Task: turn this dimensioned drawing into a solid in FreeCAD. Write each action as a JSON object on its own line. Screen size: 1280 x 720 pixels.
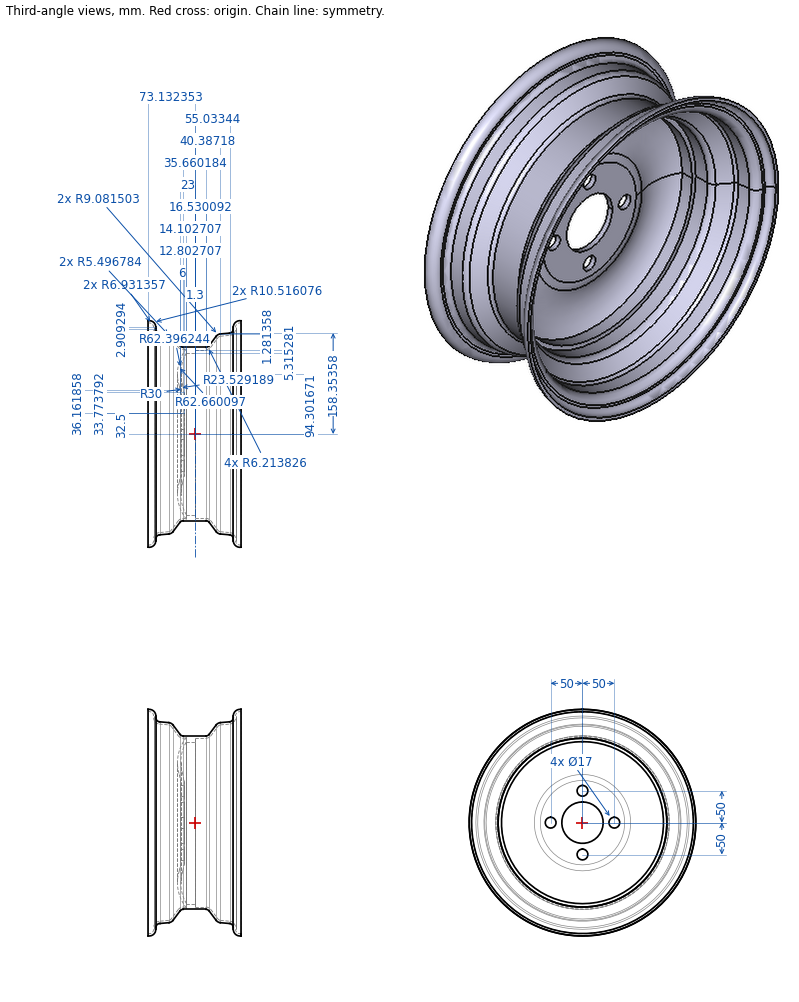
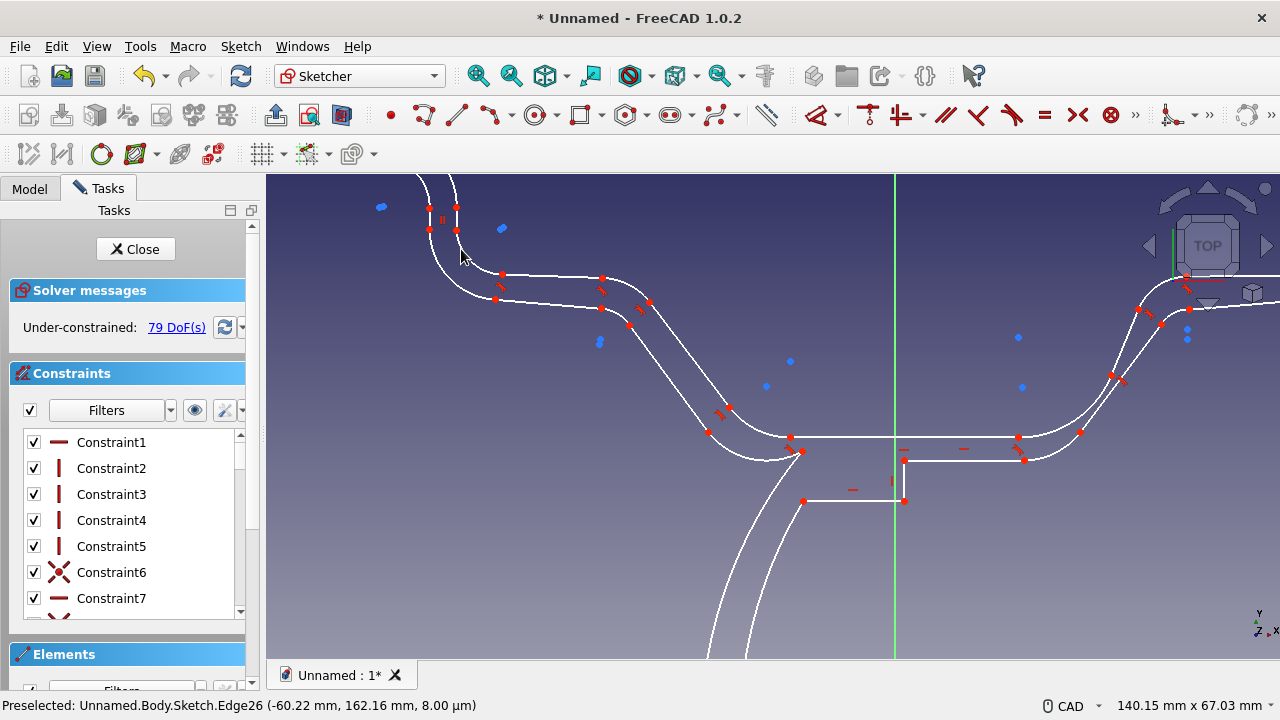
{"action": "scroll", "coordinate": [457, 219], "scroll_direction": "up", "scroll_amount": 2}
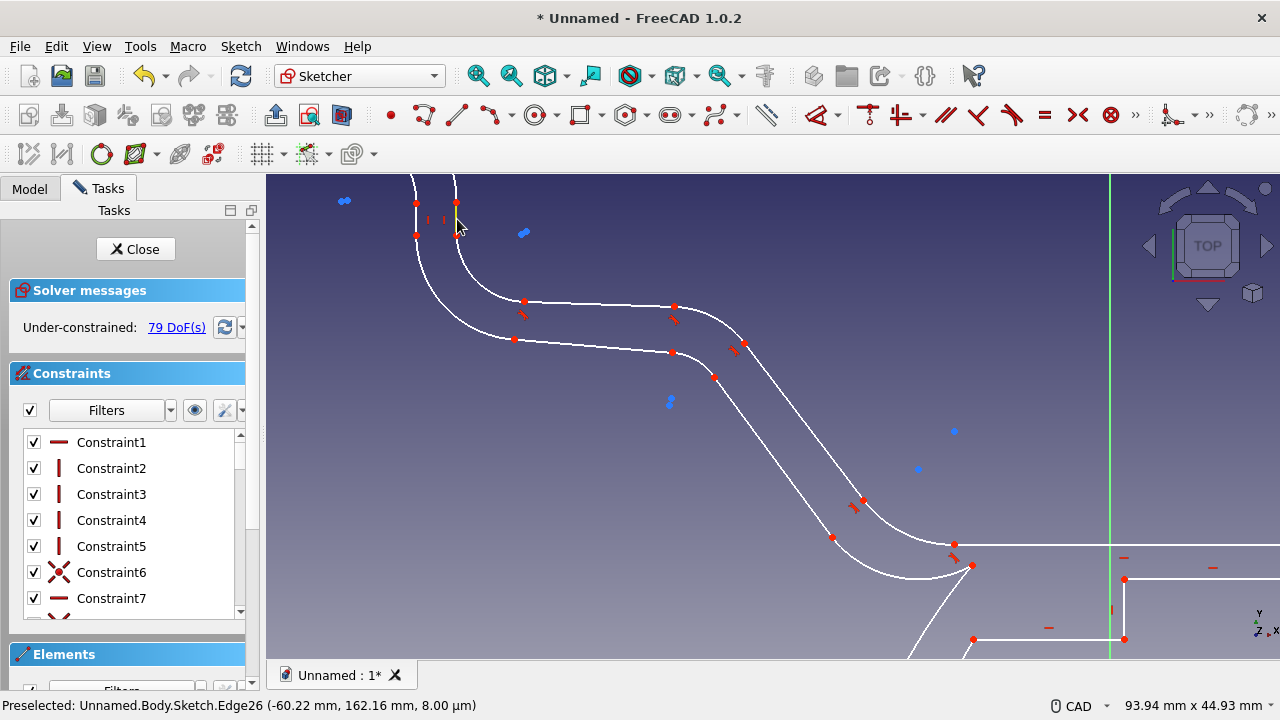
{"action": "left_click", "coordinate": [456, 219]}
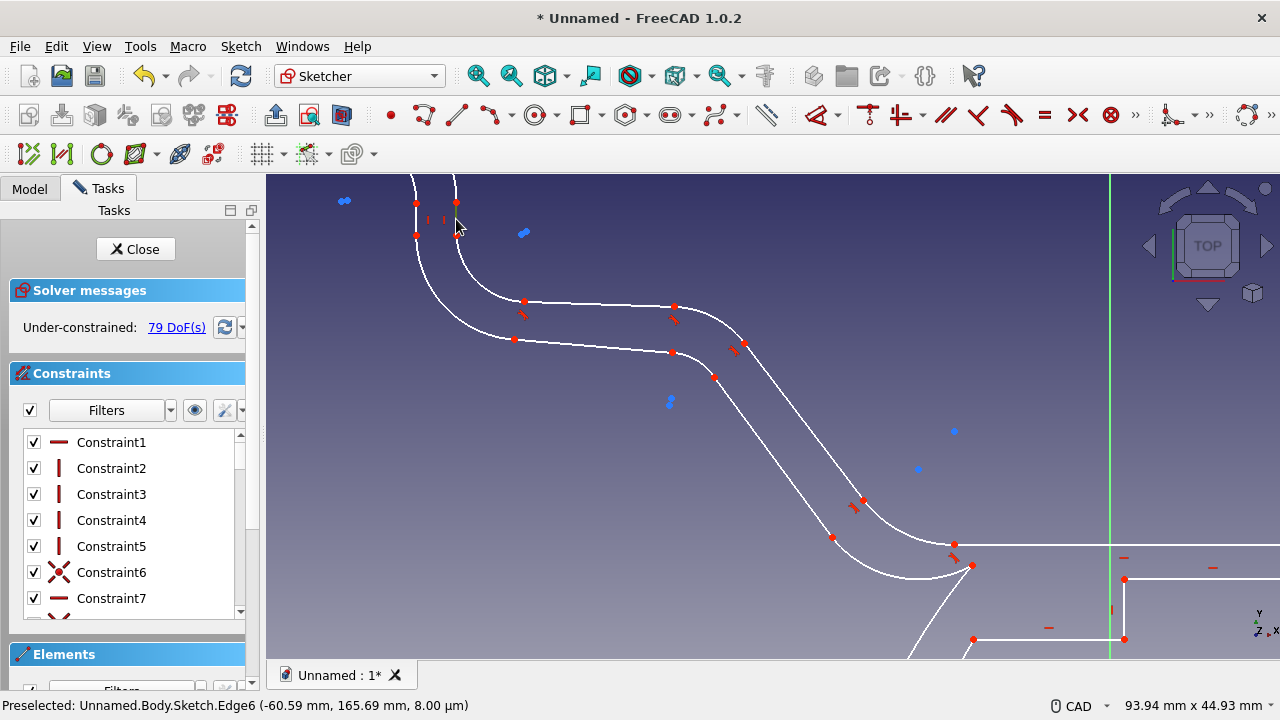
{"action": "left_click", "coordinate": [465, 265]}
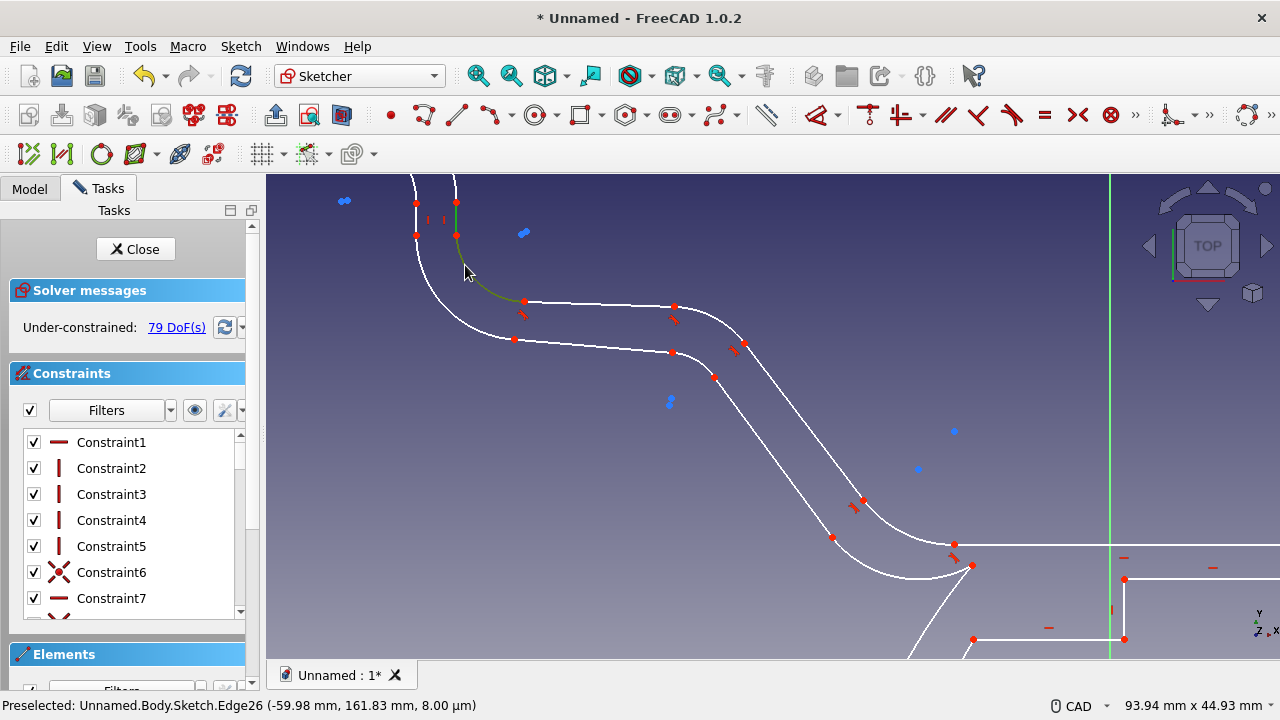
{"action": "key", "text": "t"}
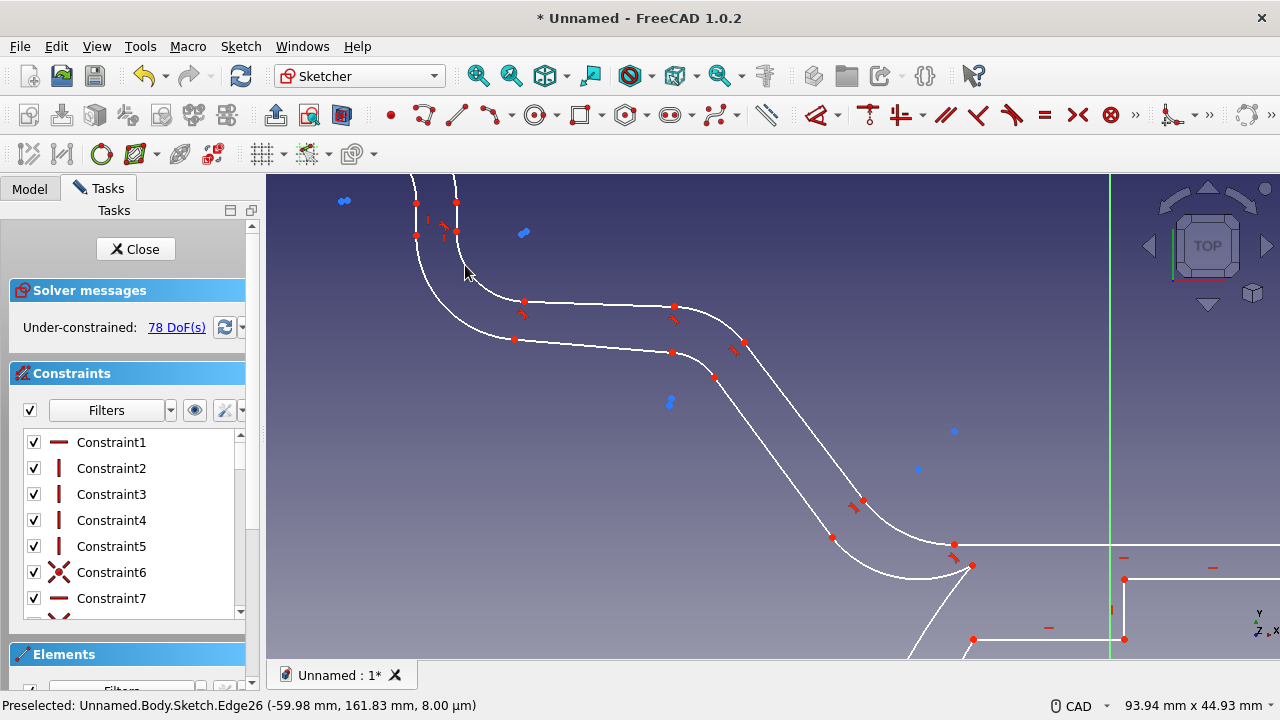
{"action": "left_click", "coordinate": [457, 220]}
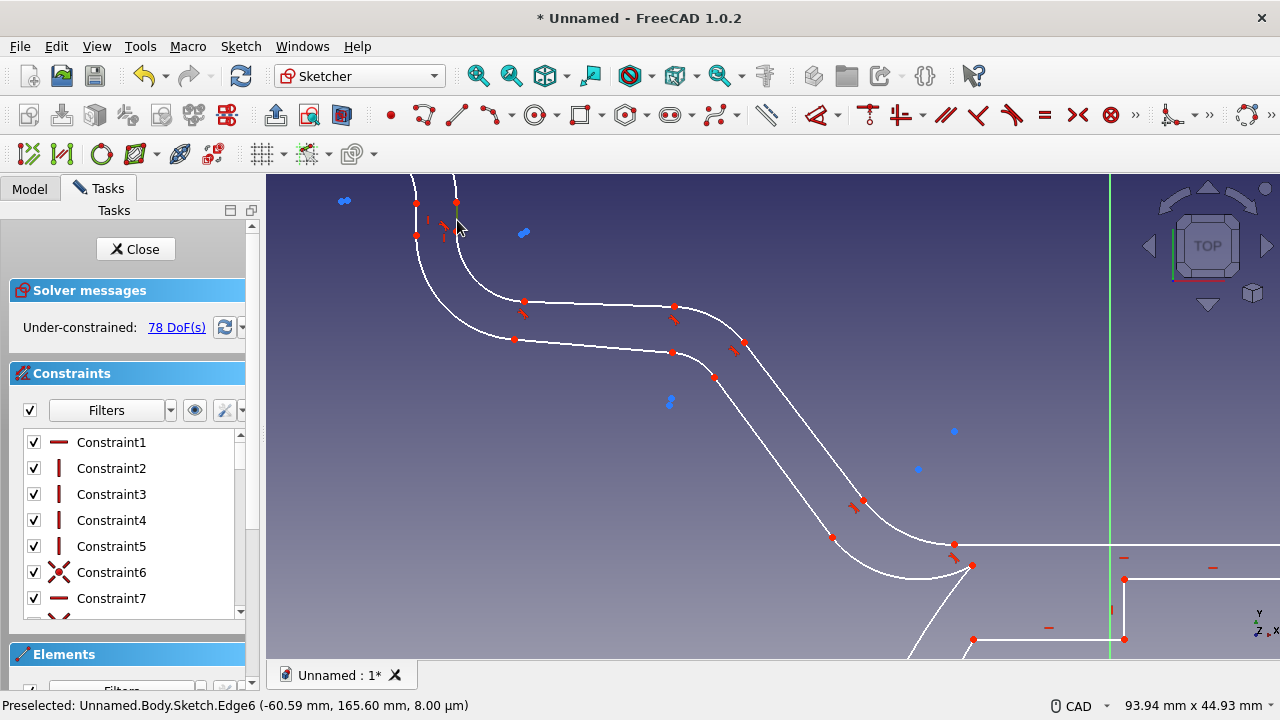
{"action": "scroll", "coordinate": [624, 291], "scroll_direction": "down", "scroll_amount": 9}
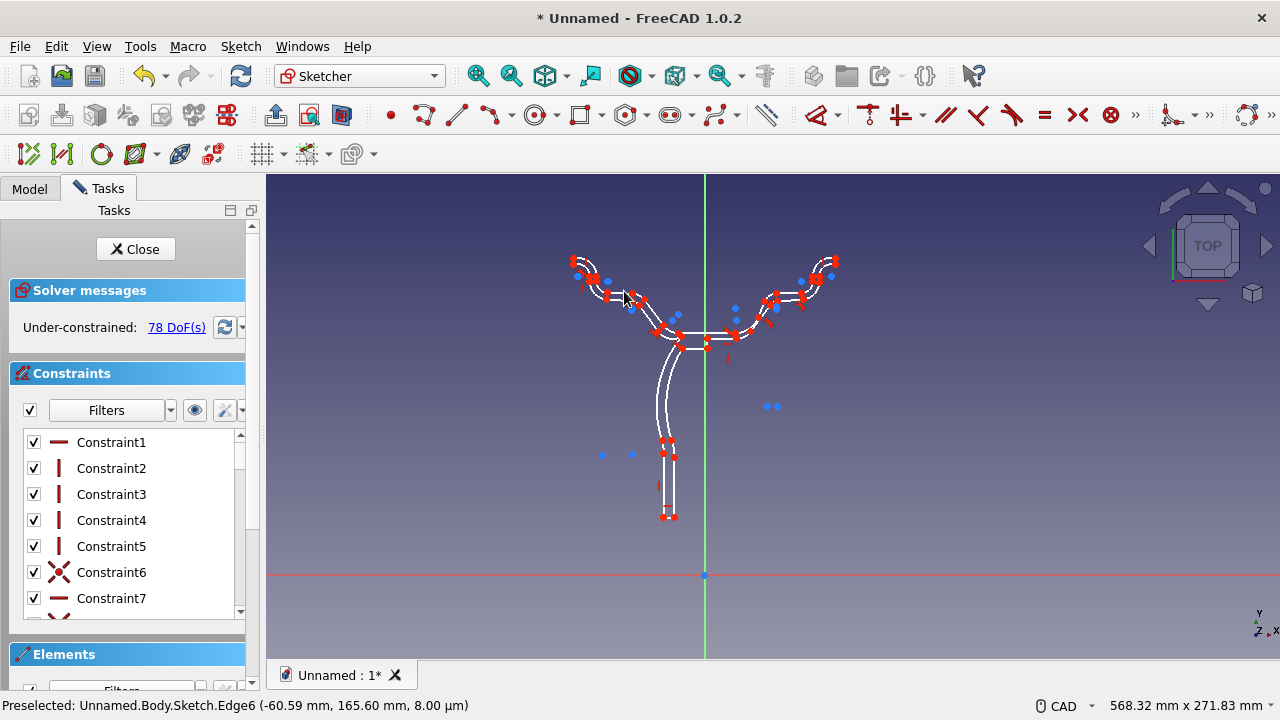
{"action": "scroll", "coordinate": [594, 267], "scroll_direction": "up", "scroll_amount": 4}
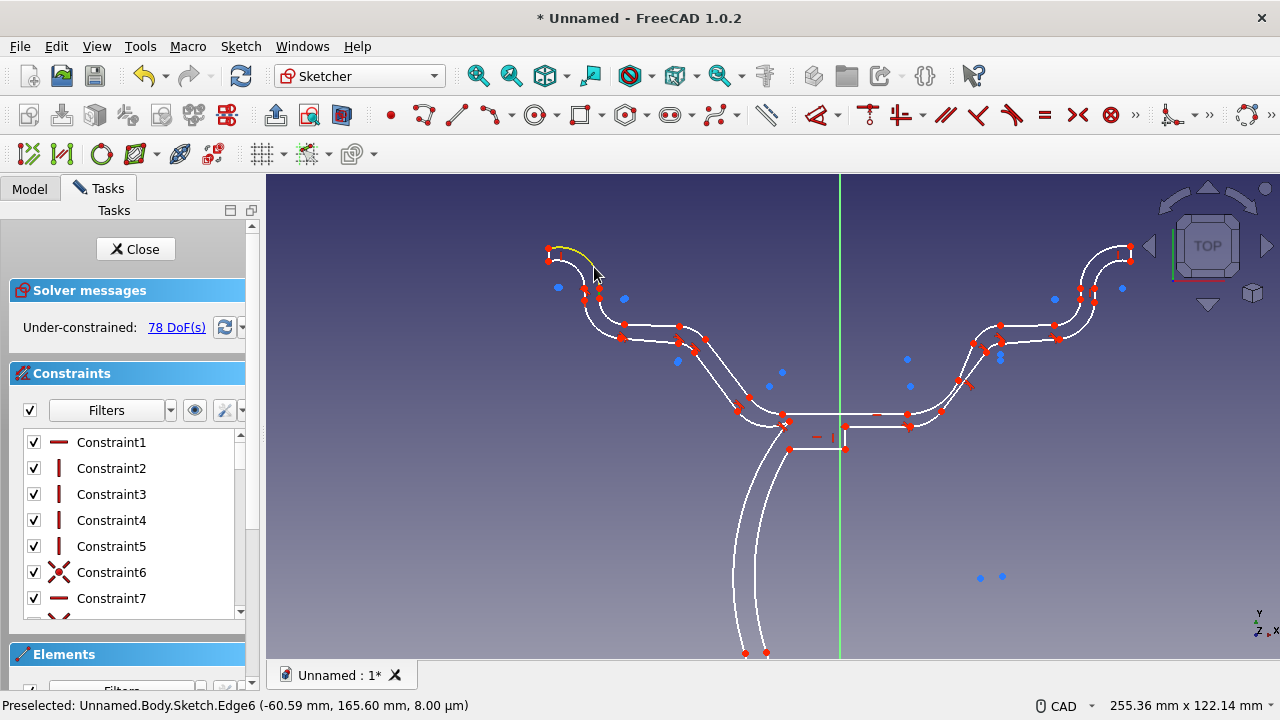
{"action": "left_click", "coordinate": [594, 267]}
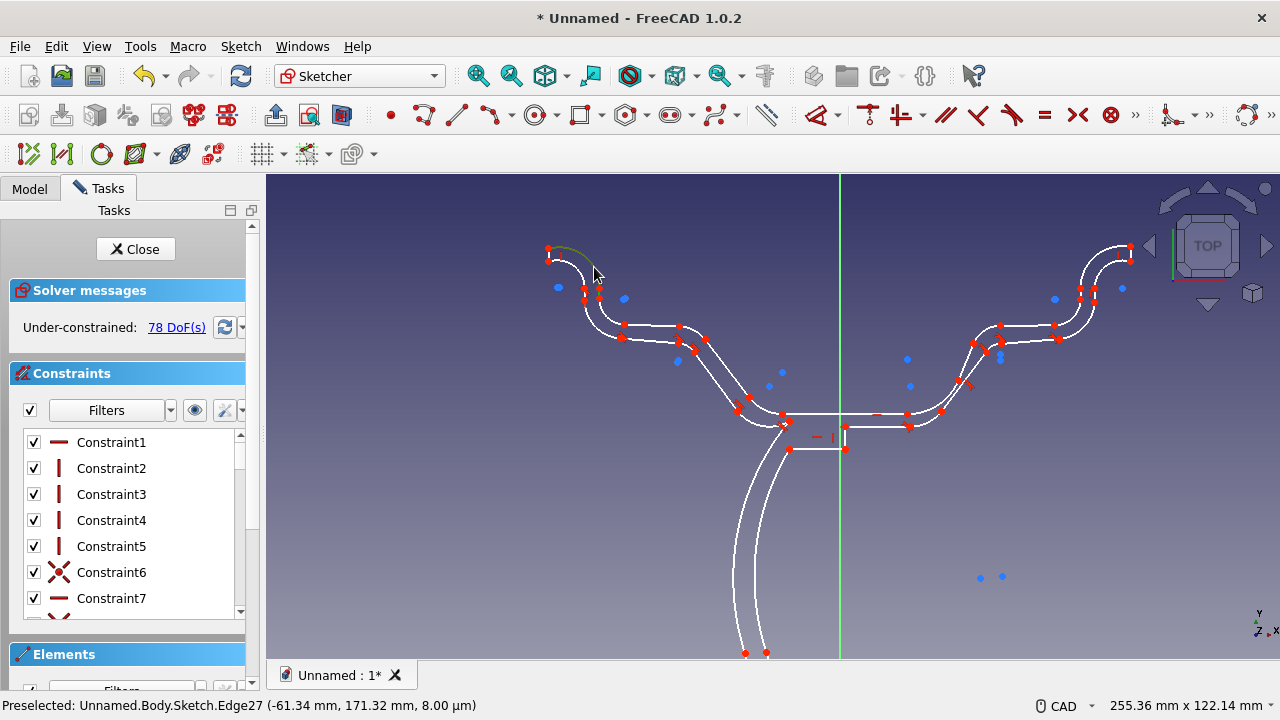
{"action": "left_click", "coordinate": [1012, 116]}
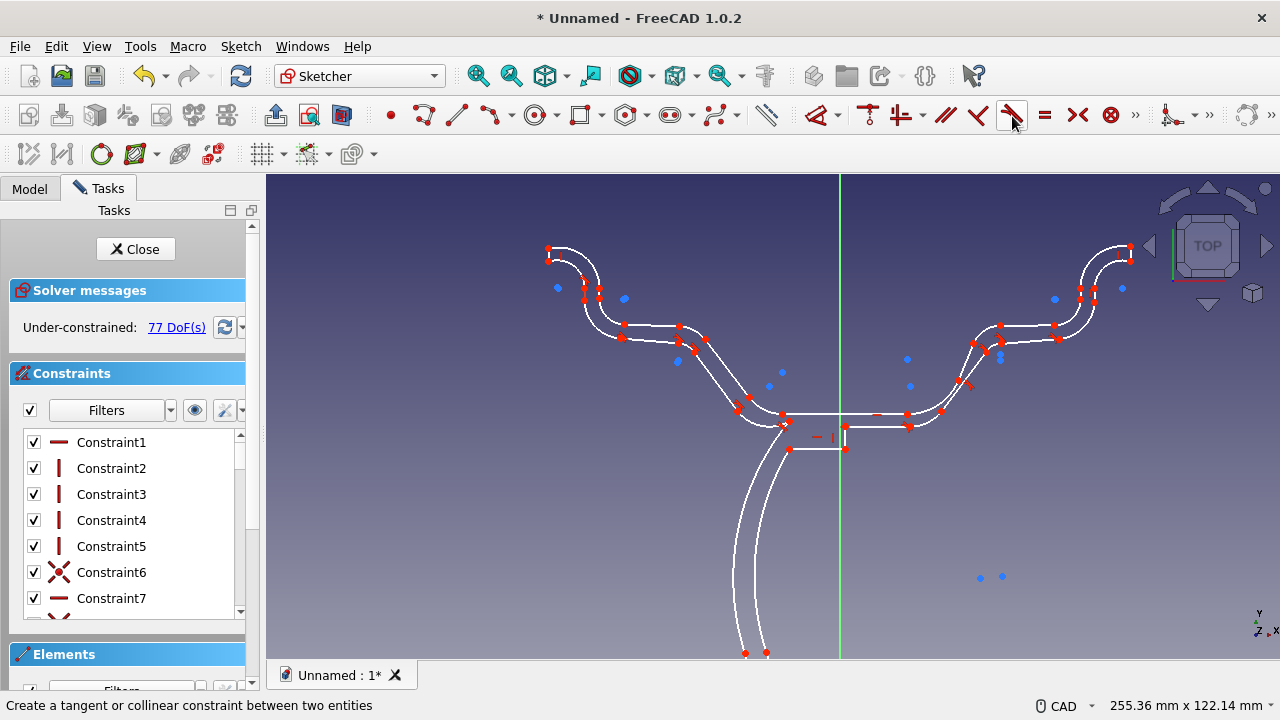
{"action": "scroll", "coordinate": [585, 294], "scroll_direction": "up", "scroll_amount": 5}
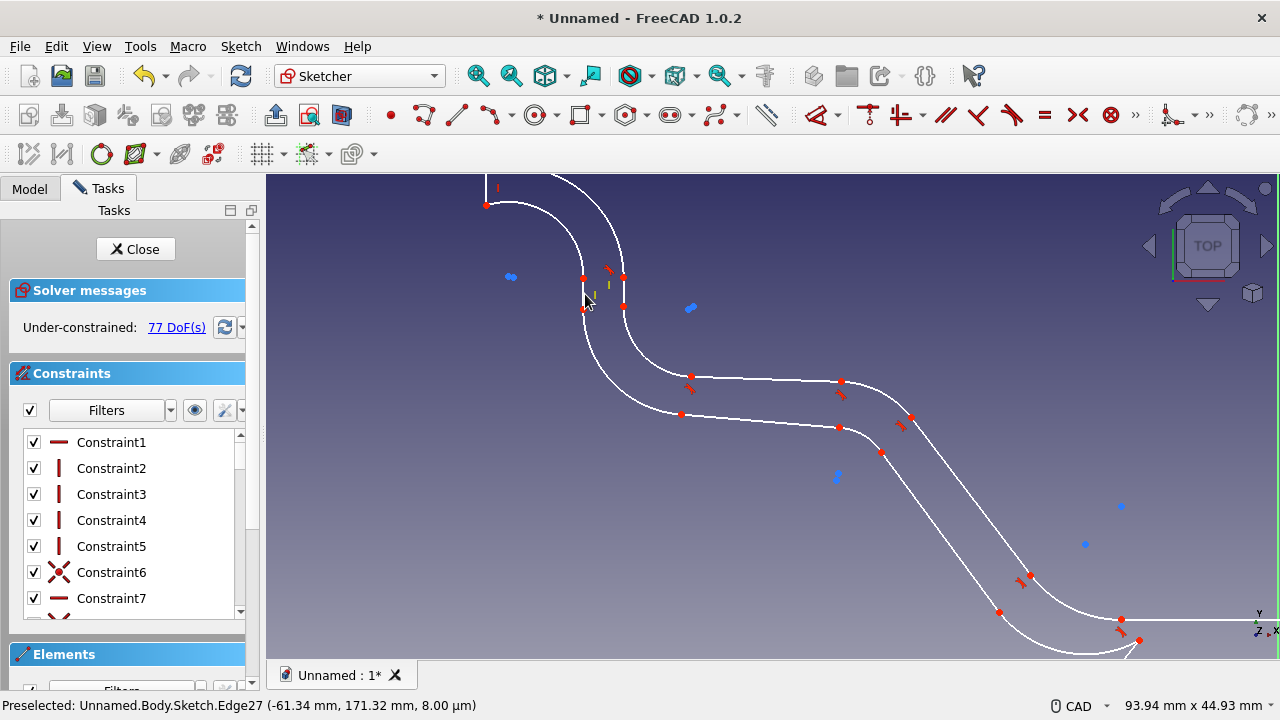
{"action": "left_click", "coordinate": [583, 294]}